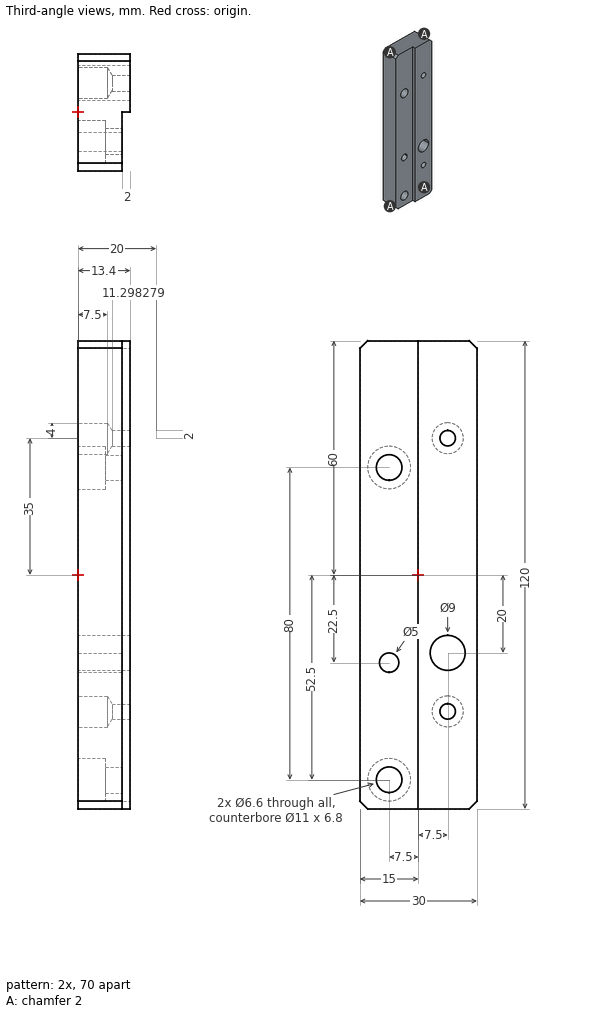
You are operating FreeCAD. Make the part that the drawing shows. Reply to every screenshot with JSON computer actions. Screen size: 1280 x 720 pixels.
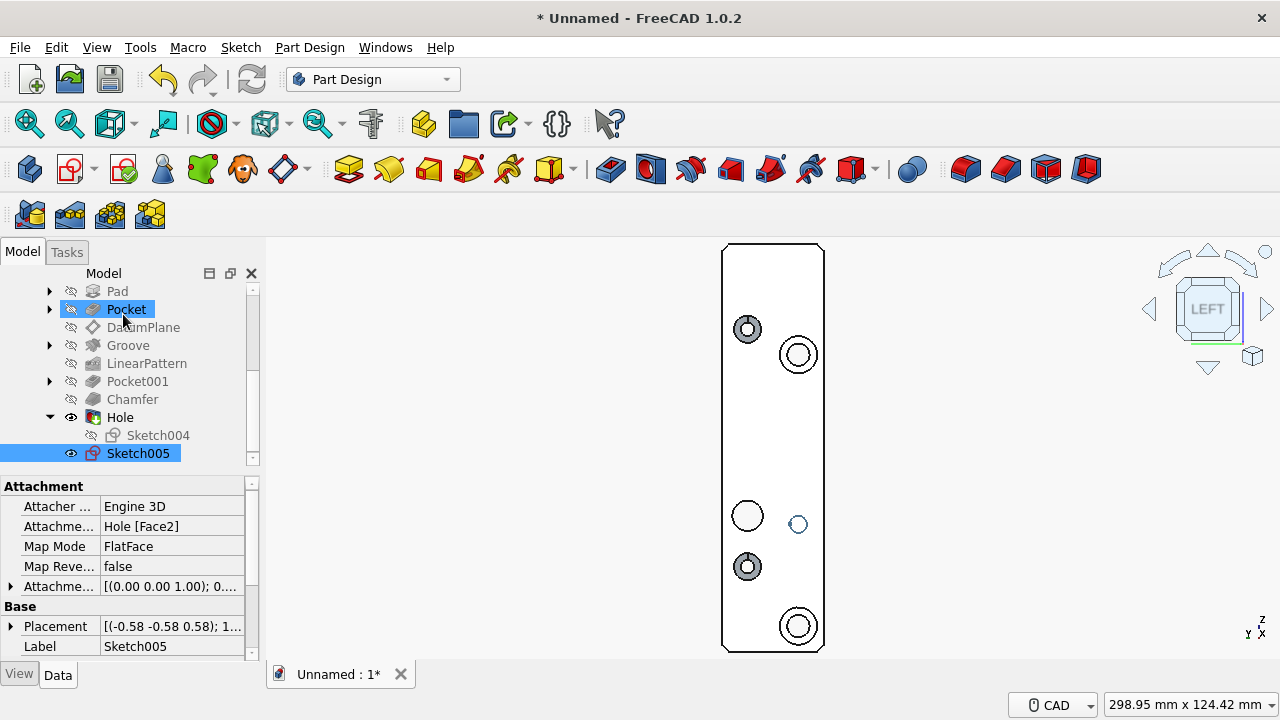
{"action": "left_click", "coordinate": [612, 170]}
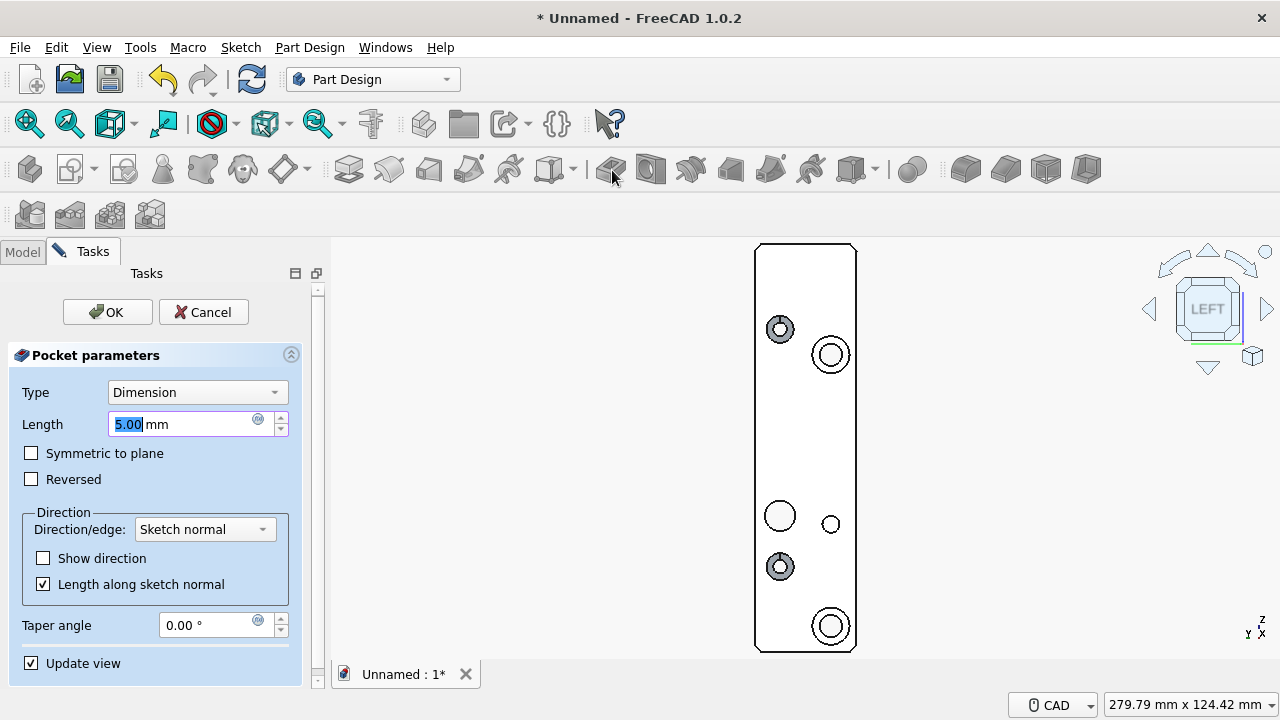
{"action": "left_click", "coordinate": [198, 392]}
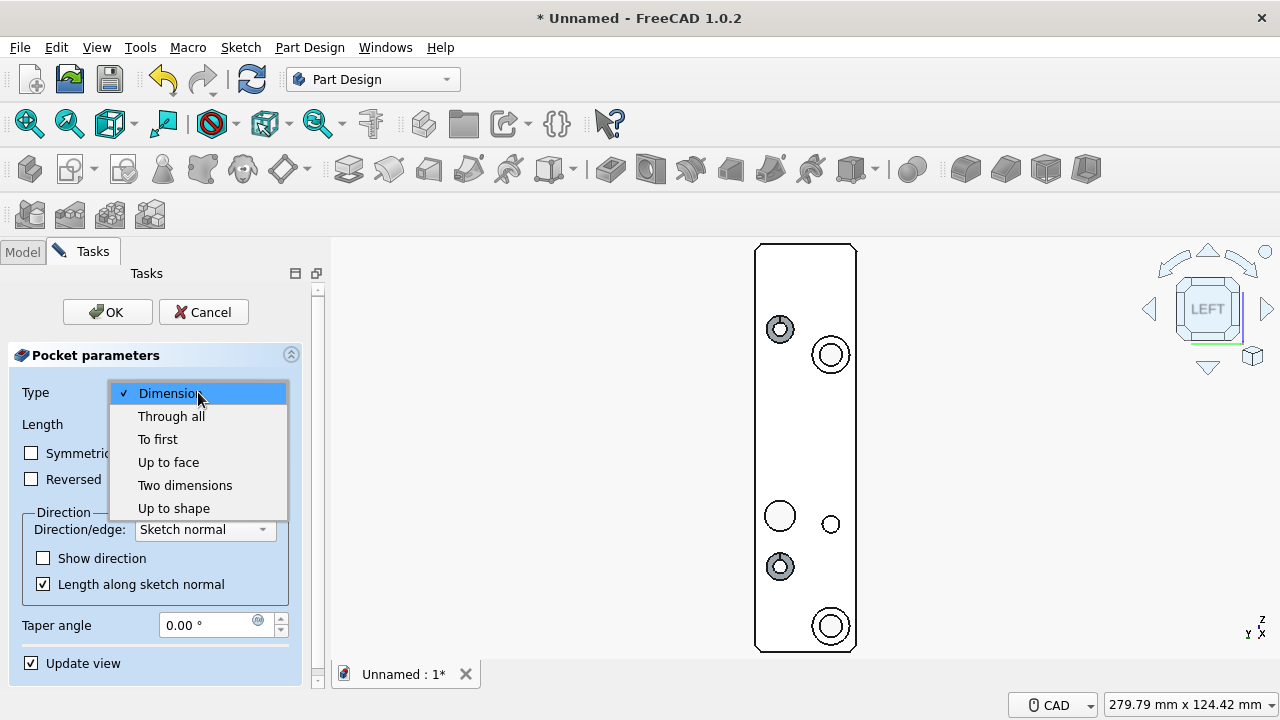
{"action": "left_click", "coordinate": [198, 416]}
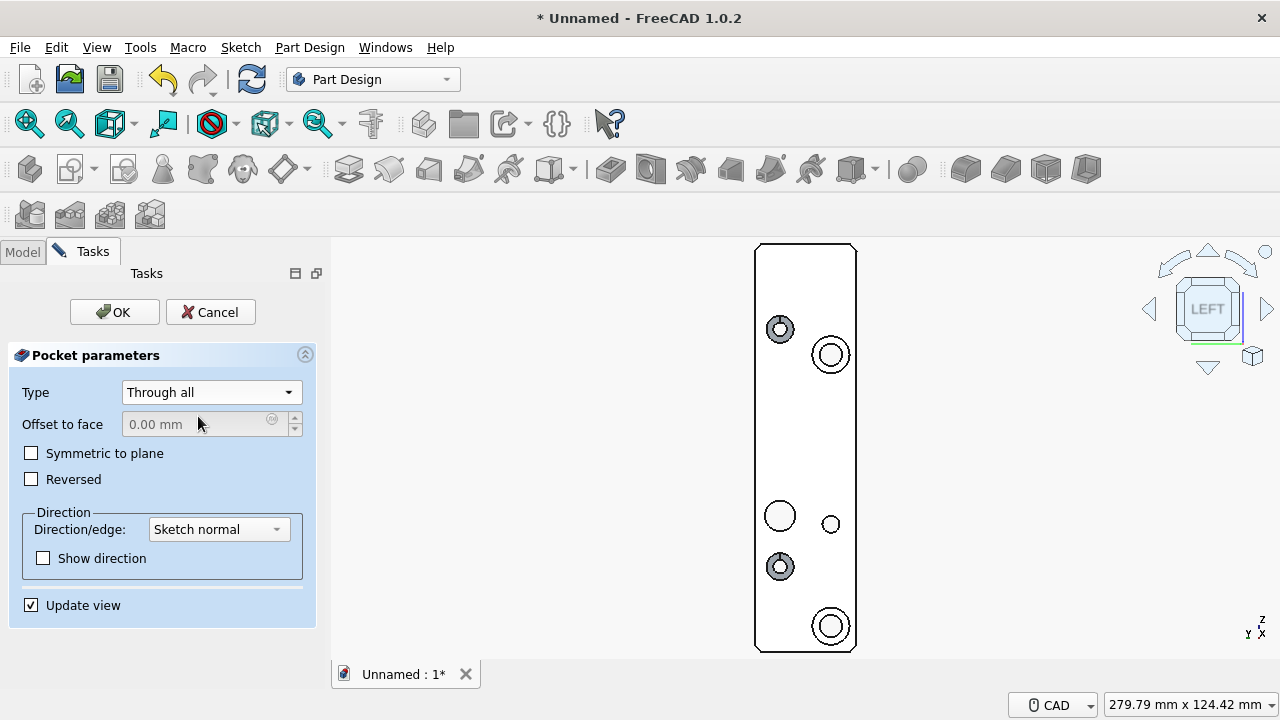
{"action": "left_click", "coordinate": [115, 312]}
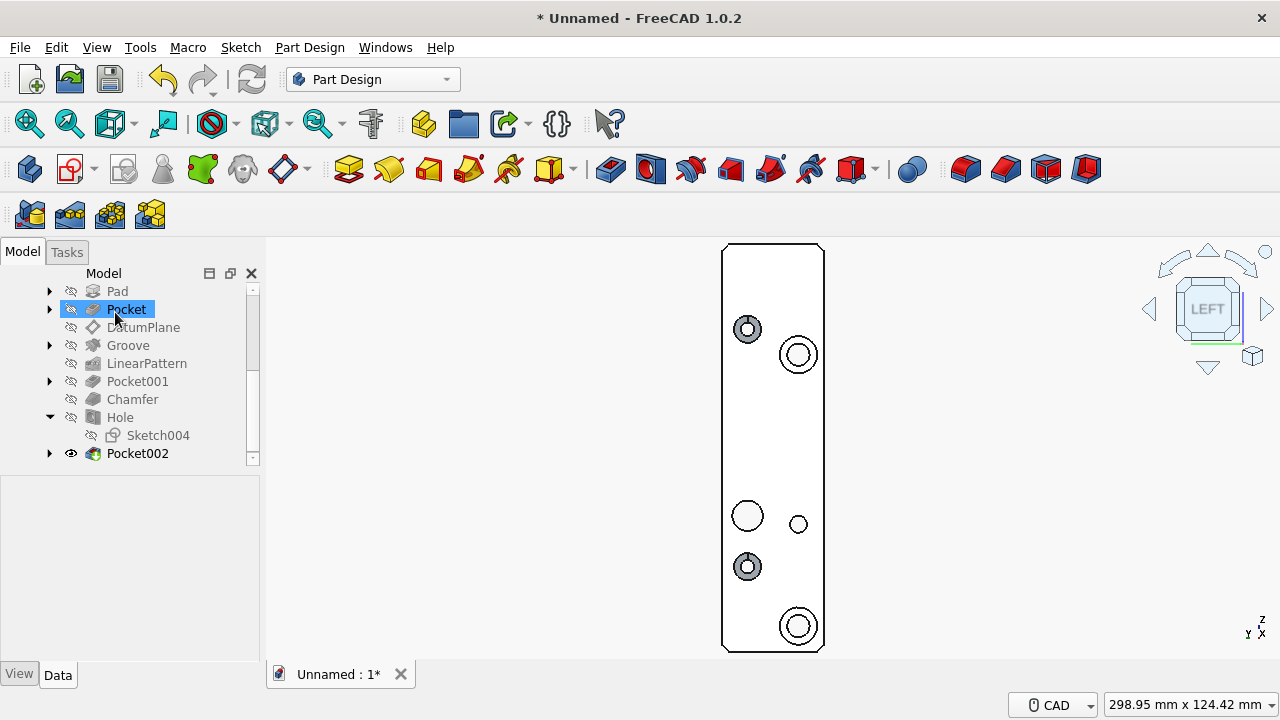
{"action": "key", "text": "0"}